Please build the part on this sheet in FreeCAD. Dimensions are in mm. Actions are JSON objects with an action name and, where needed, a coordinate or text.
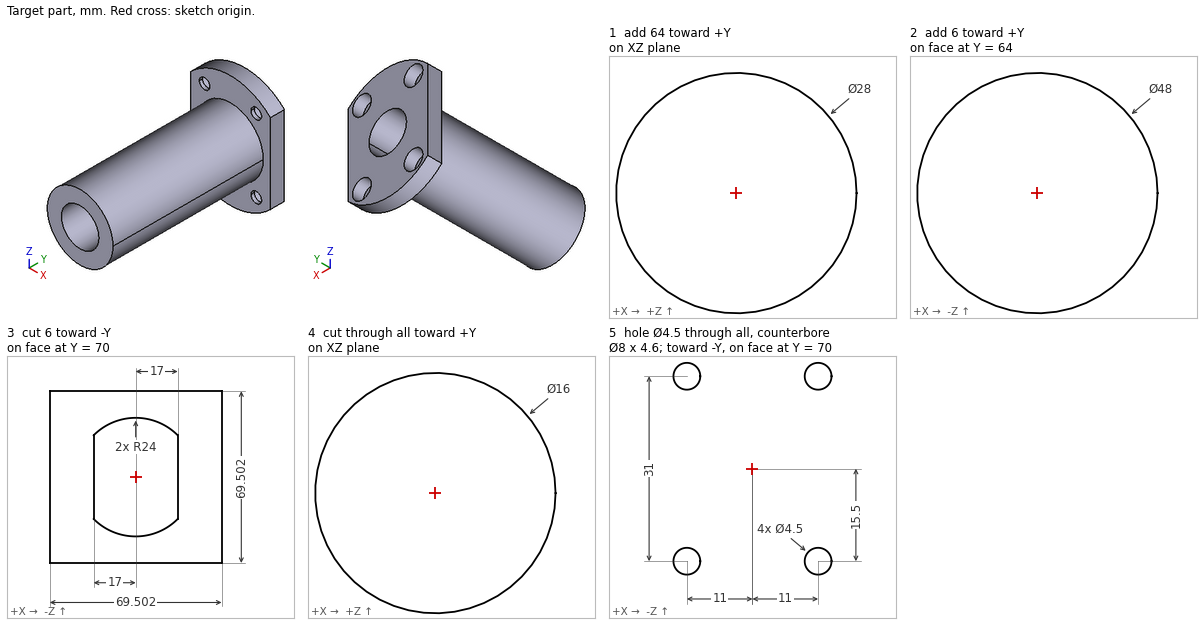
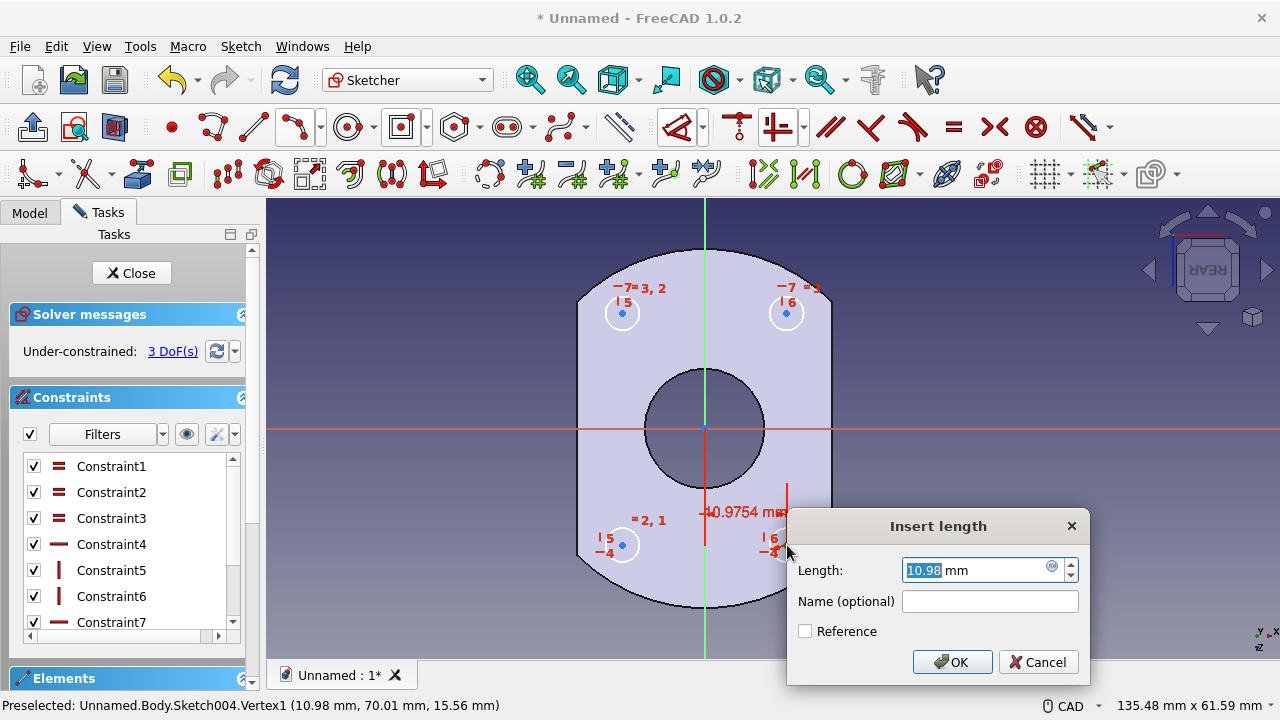
{"action": "type", "text": "11"}
{"action": "key", "text": "Return"}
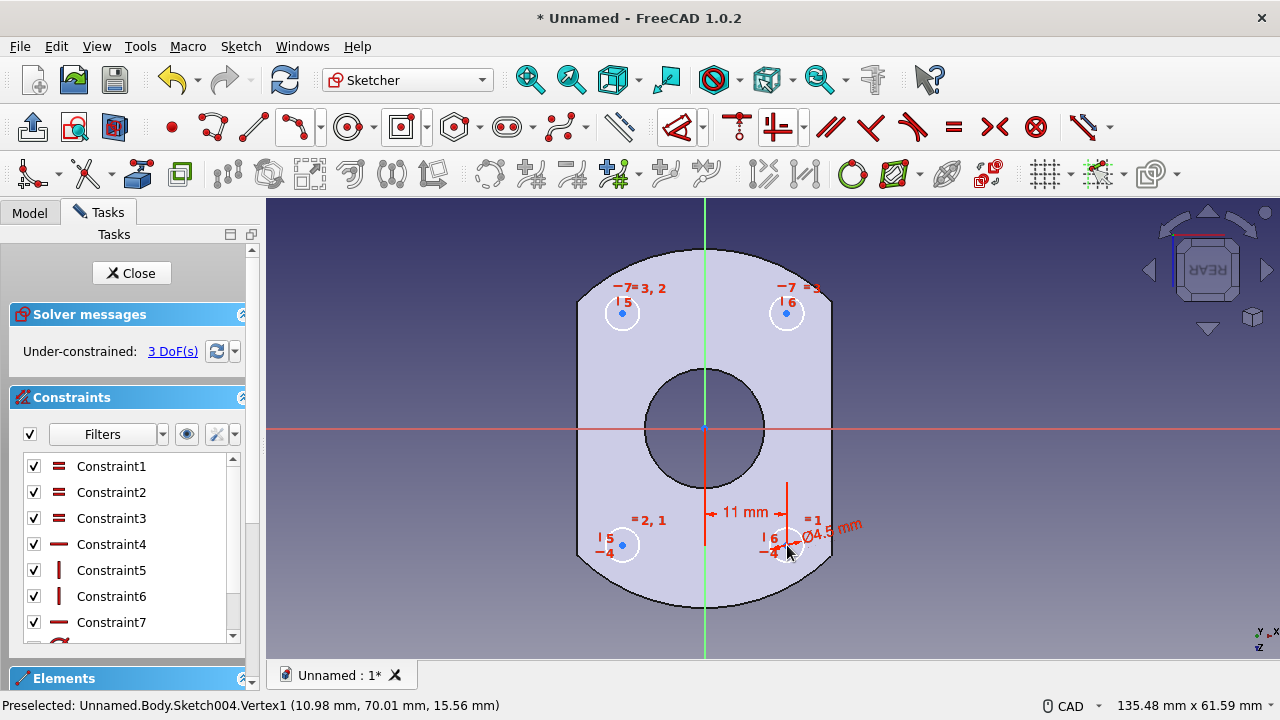
{"action": "left_click", "coordinate": [622, 545]}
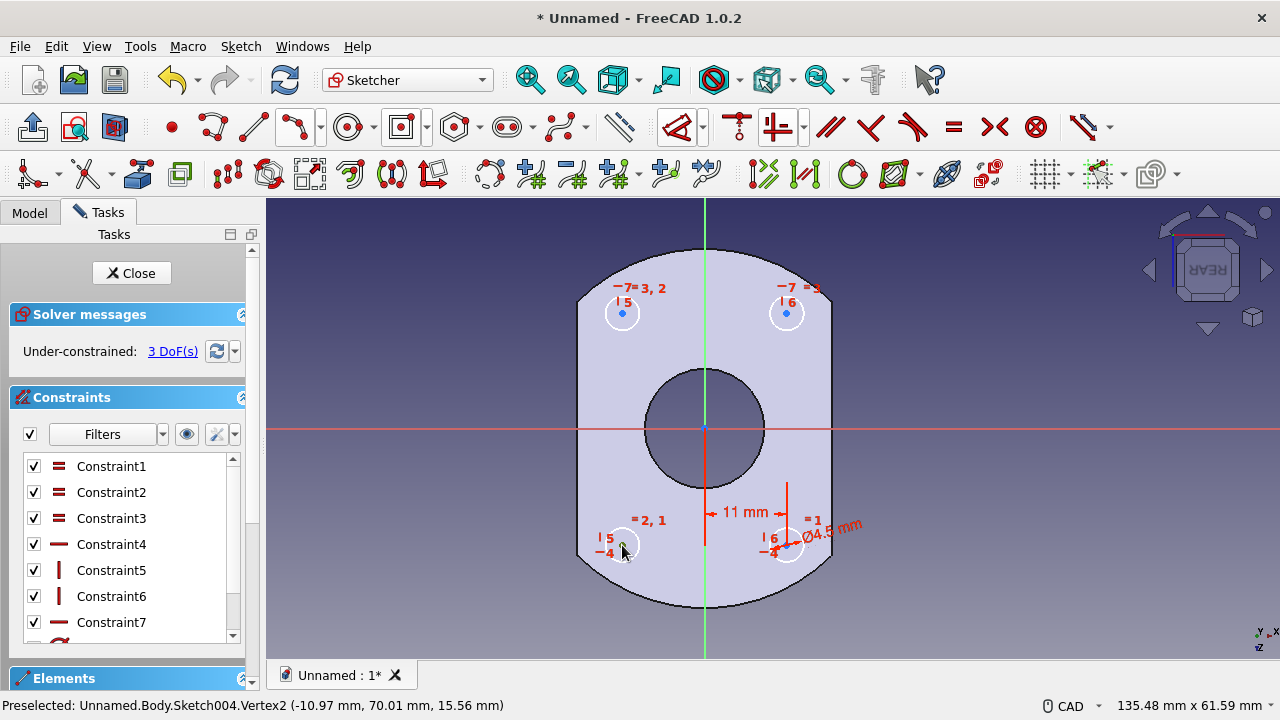
{"action": "key", "text": "l"}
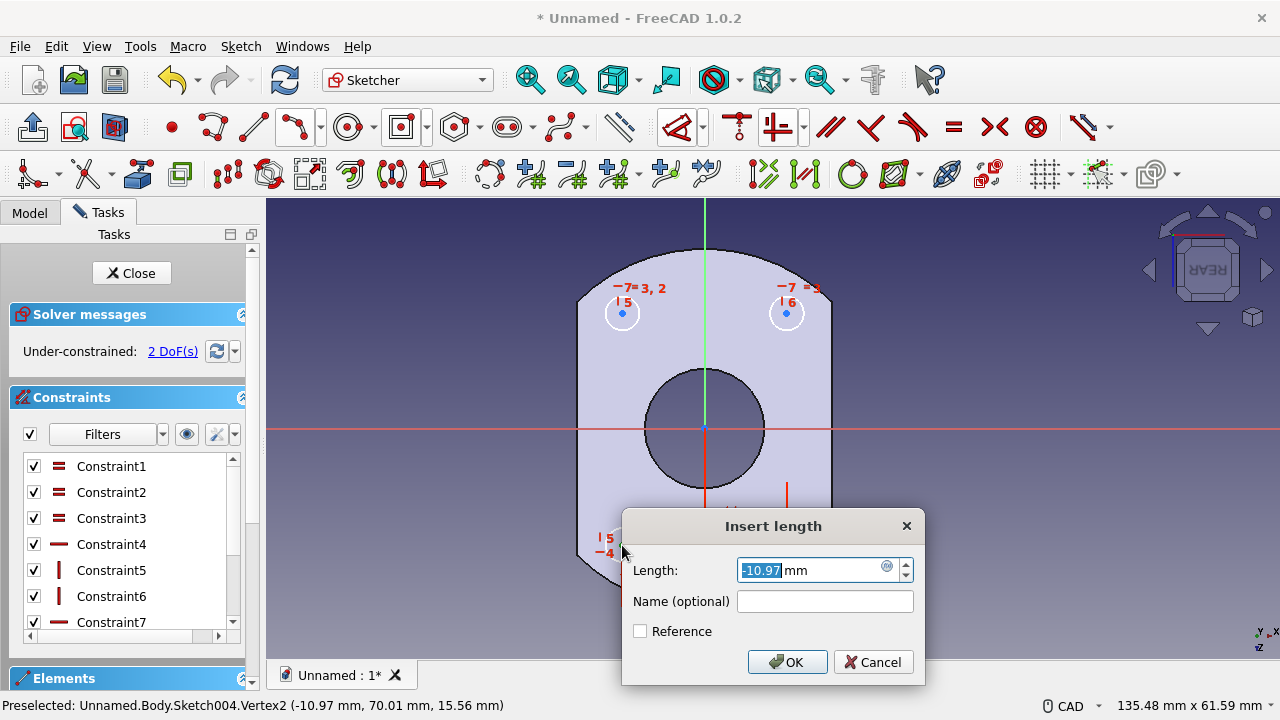
{"action": "type", "text": "-11"}
{"action": "key", "text": "Return"}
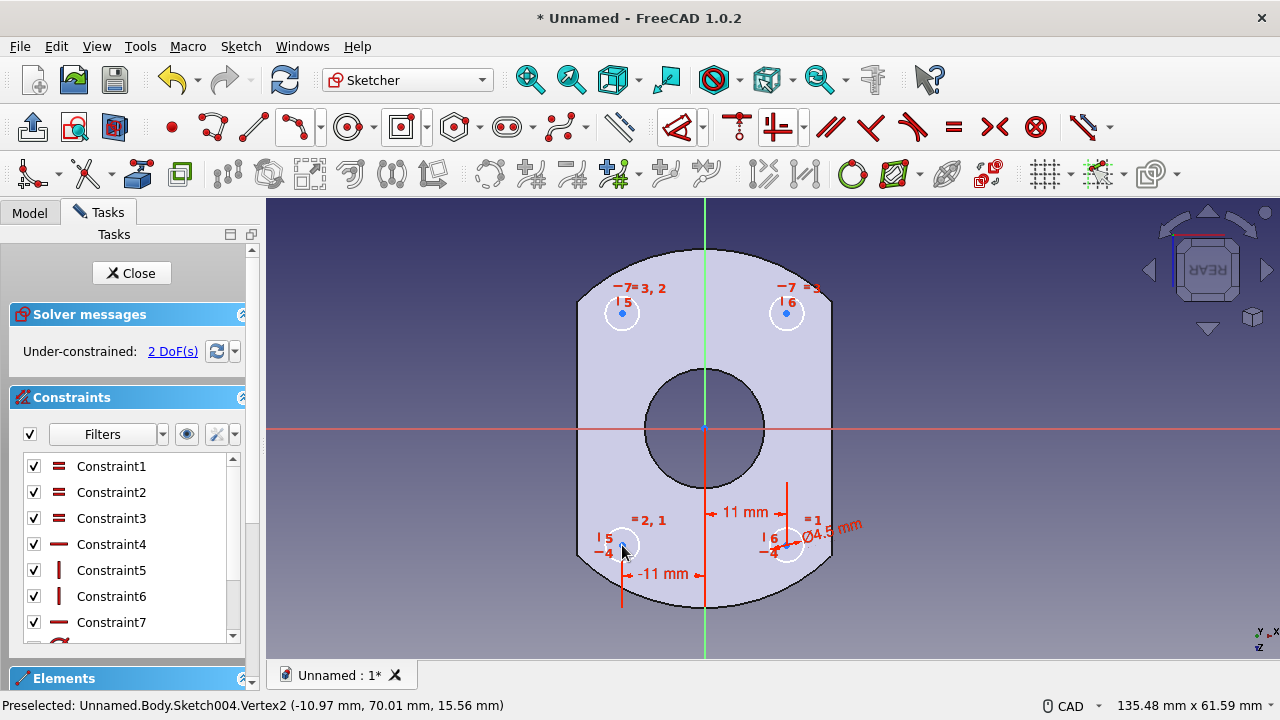
{"action": "left_click", "coordinate": [622, 545]}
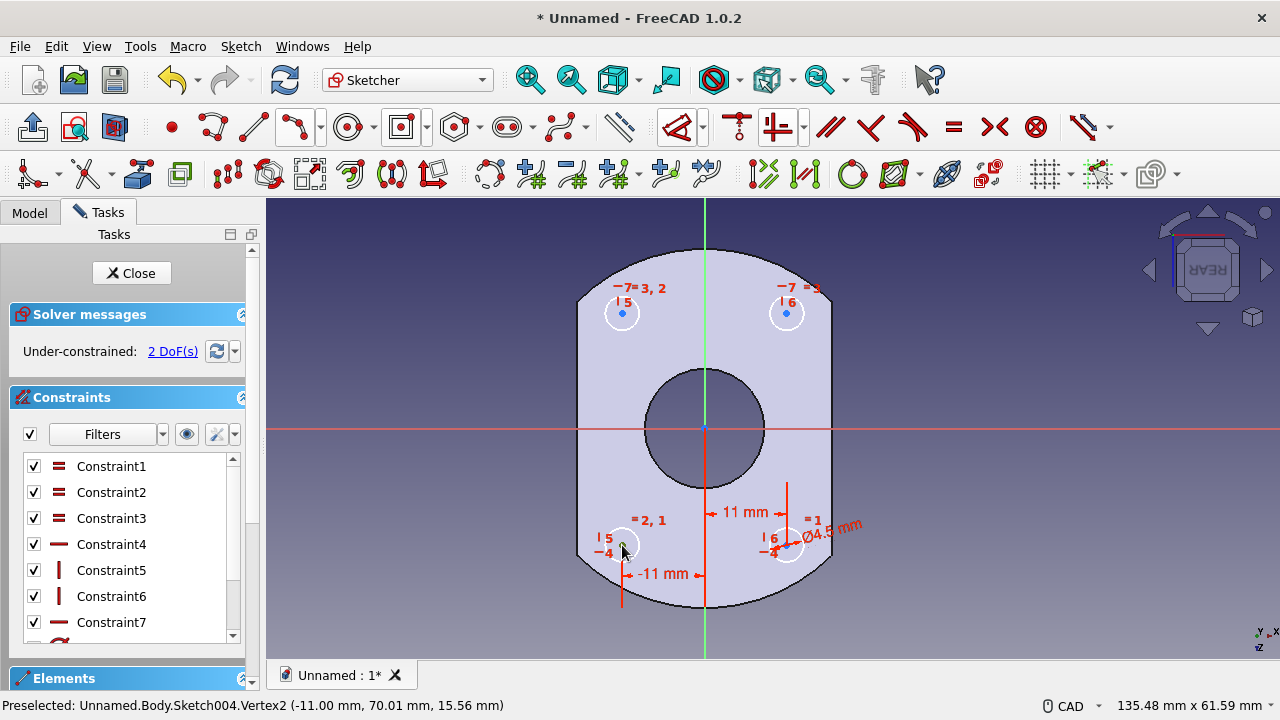
{"action": "left_click", "coordinate": [622, 313]}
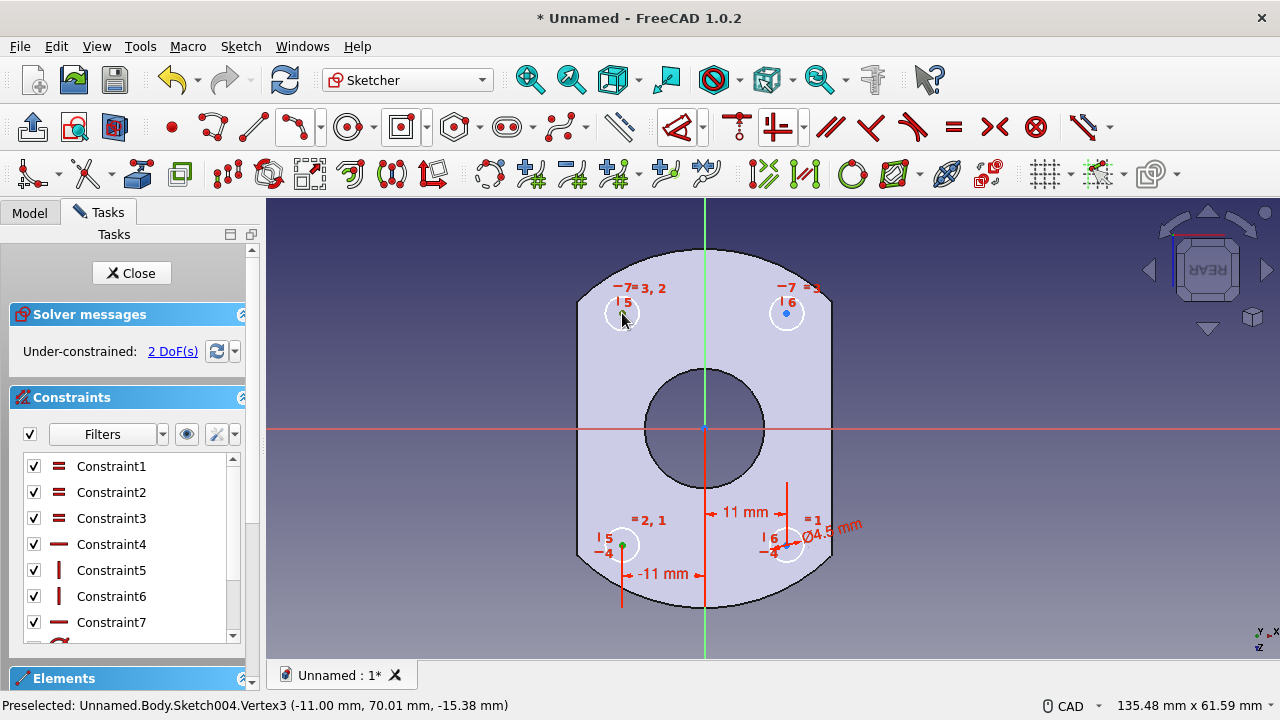
{"action": "left_click", "coordinate": [702, 128]}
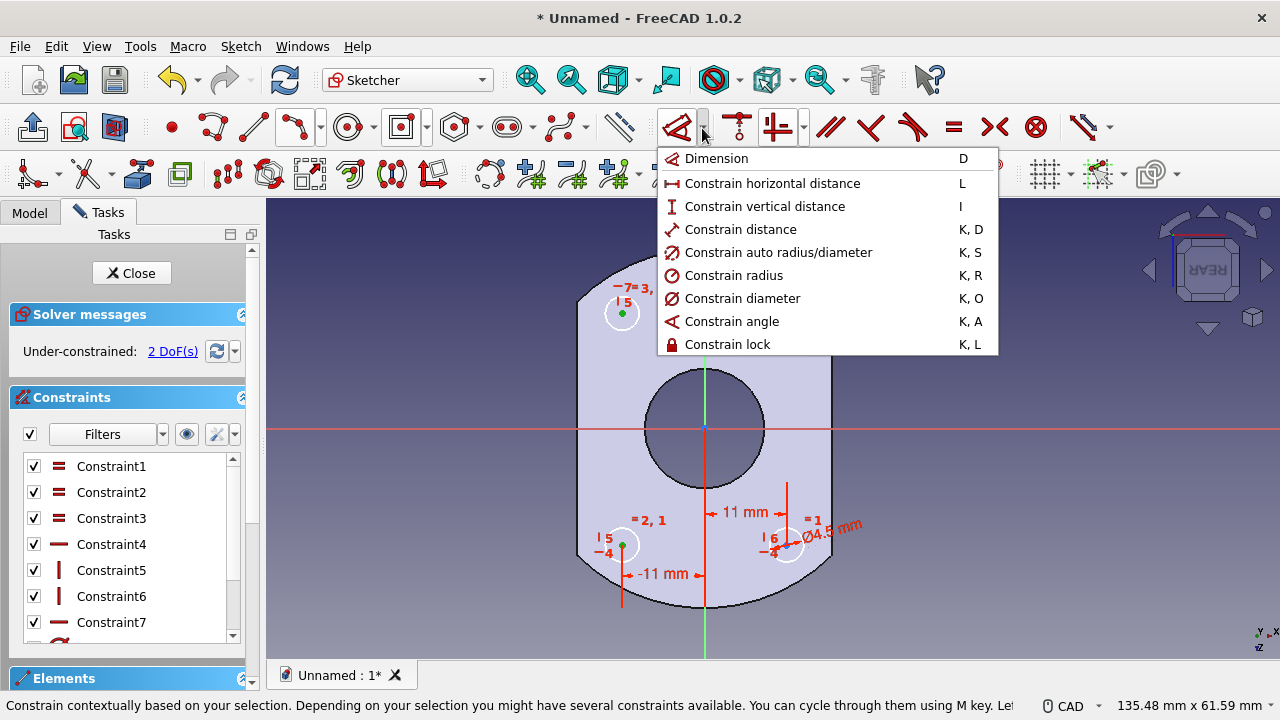
{"action": "left_click", "coordinate": [828, 206]}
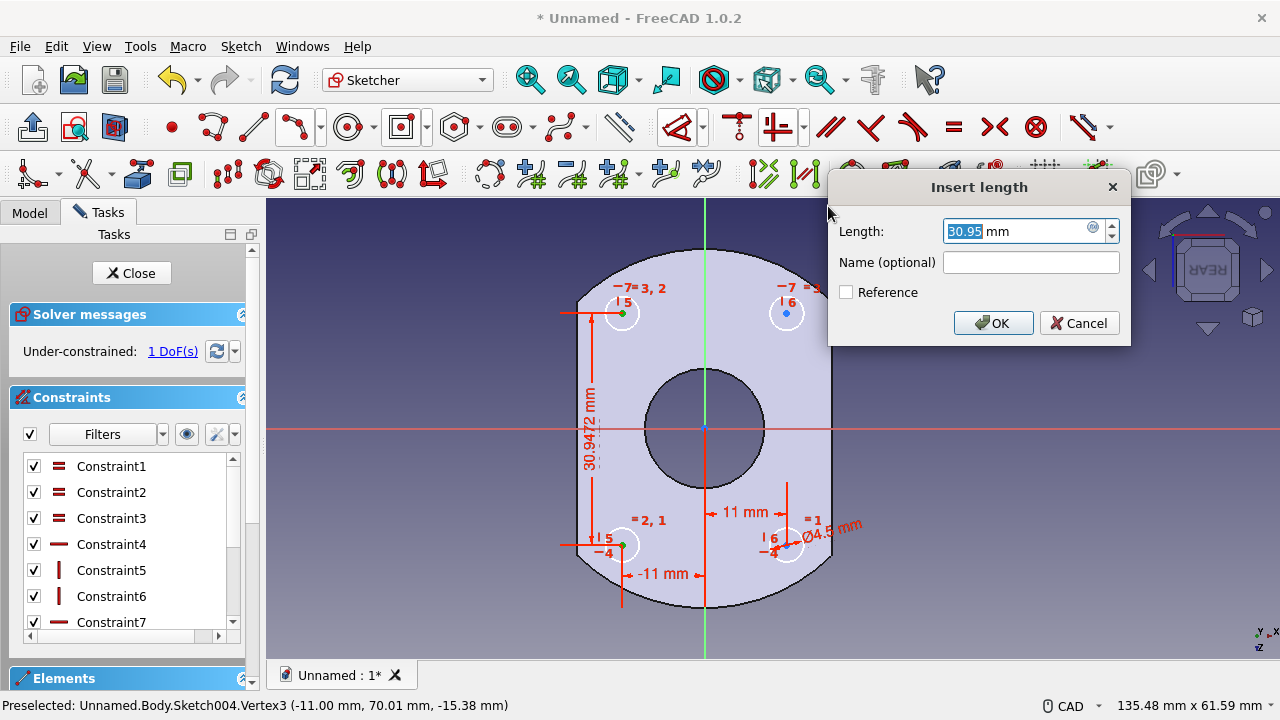
{"action": "type", "text": "31"}
{"action": "key", "text": "Return"}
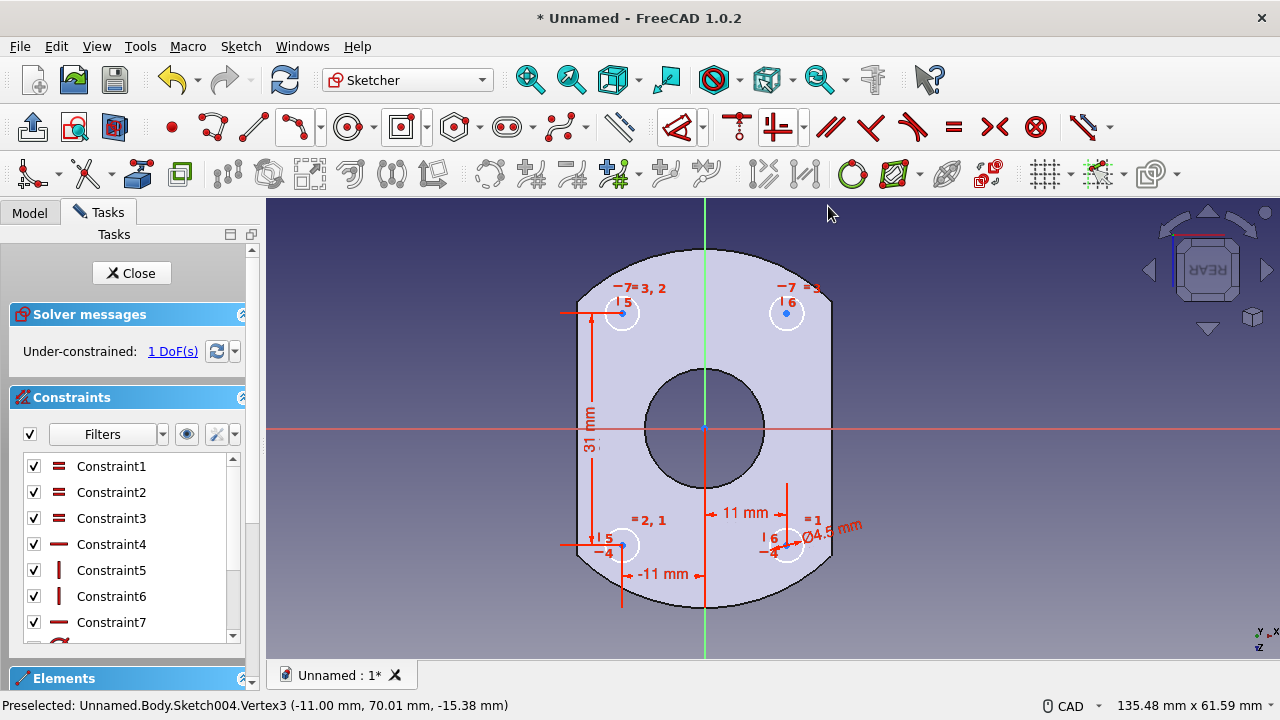
{"action": "left_click", "coordinate": [787, 545]}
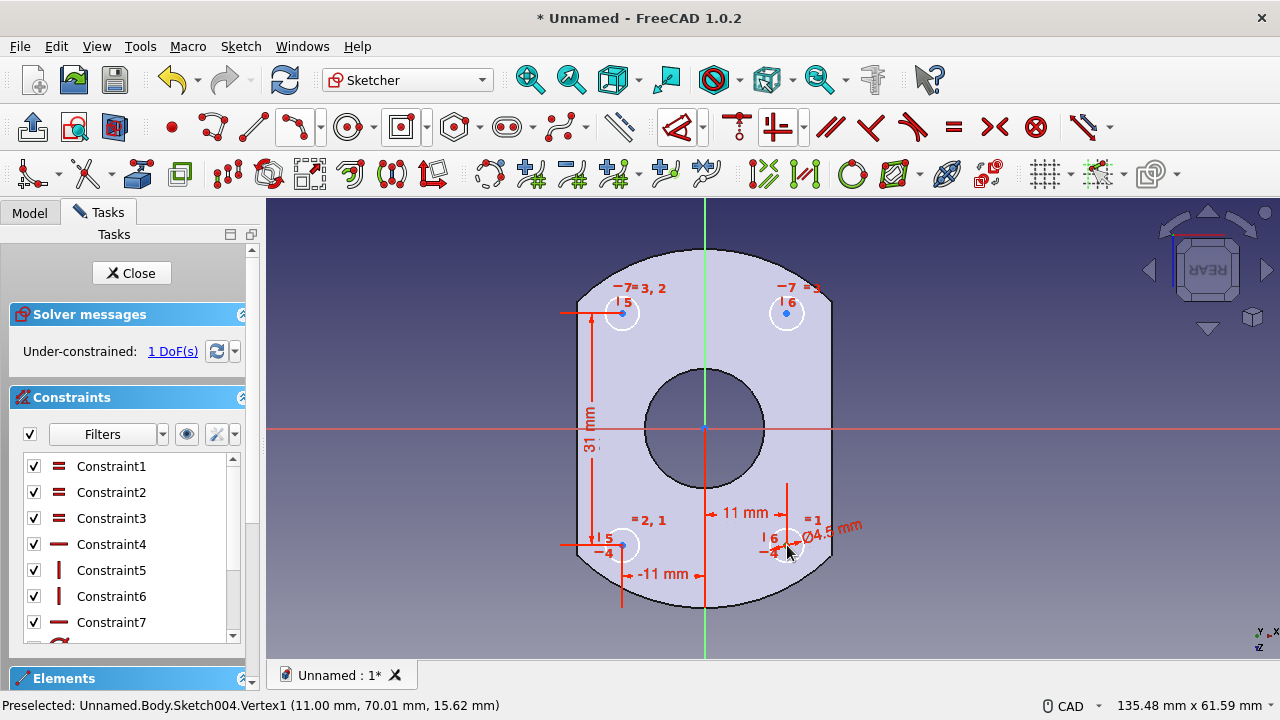
{"action": "key", "text": "i"}